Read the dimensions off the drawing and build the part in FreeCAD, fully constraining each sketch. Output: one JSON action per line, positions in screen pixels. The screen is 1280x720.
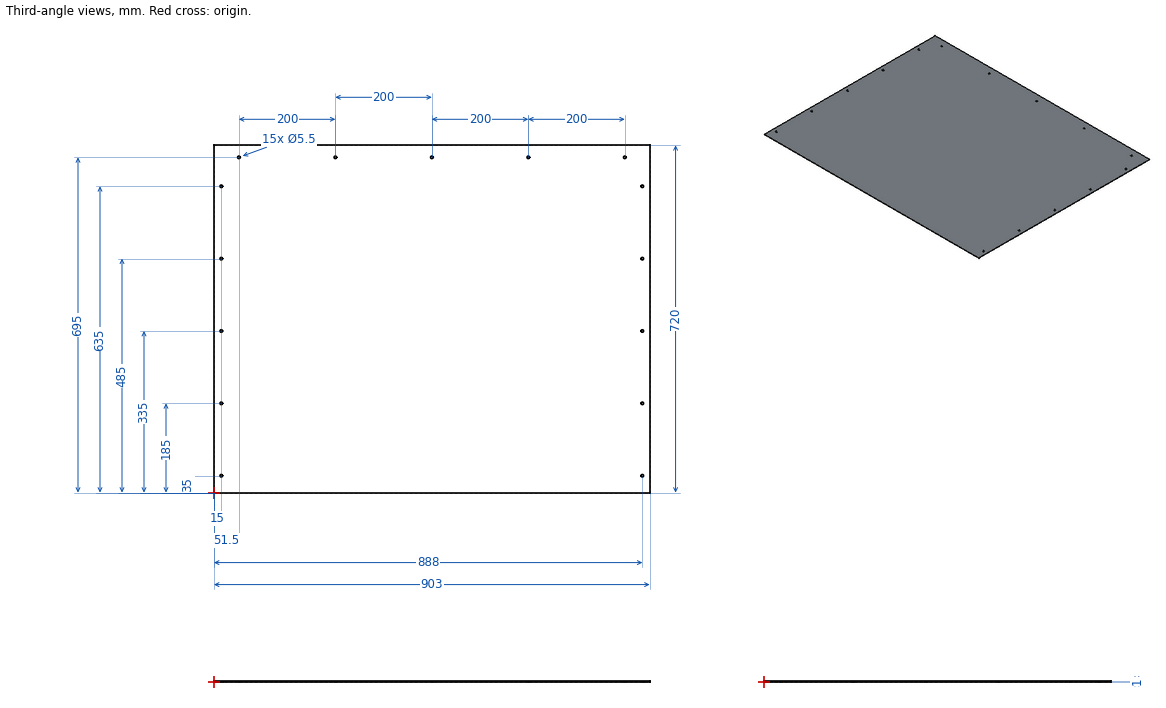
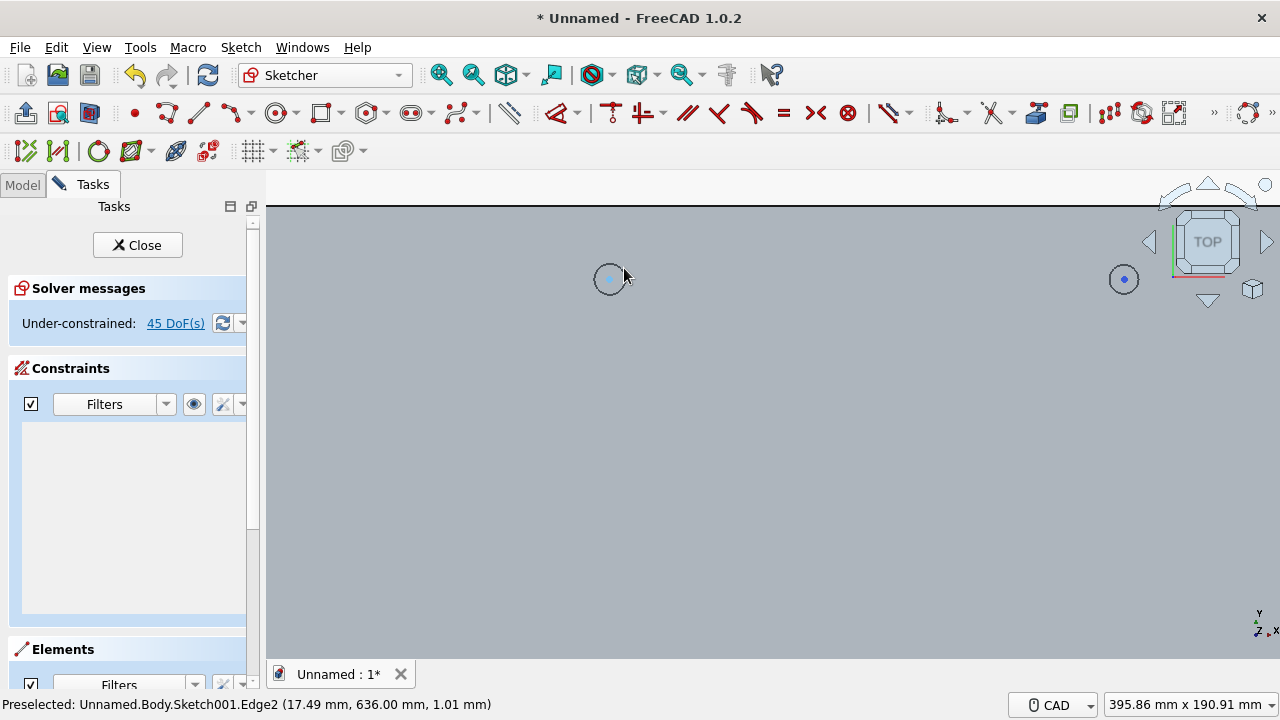
{"action": "left_click", "coordinate": [621, 268]}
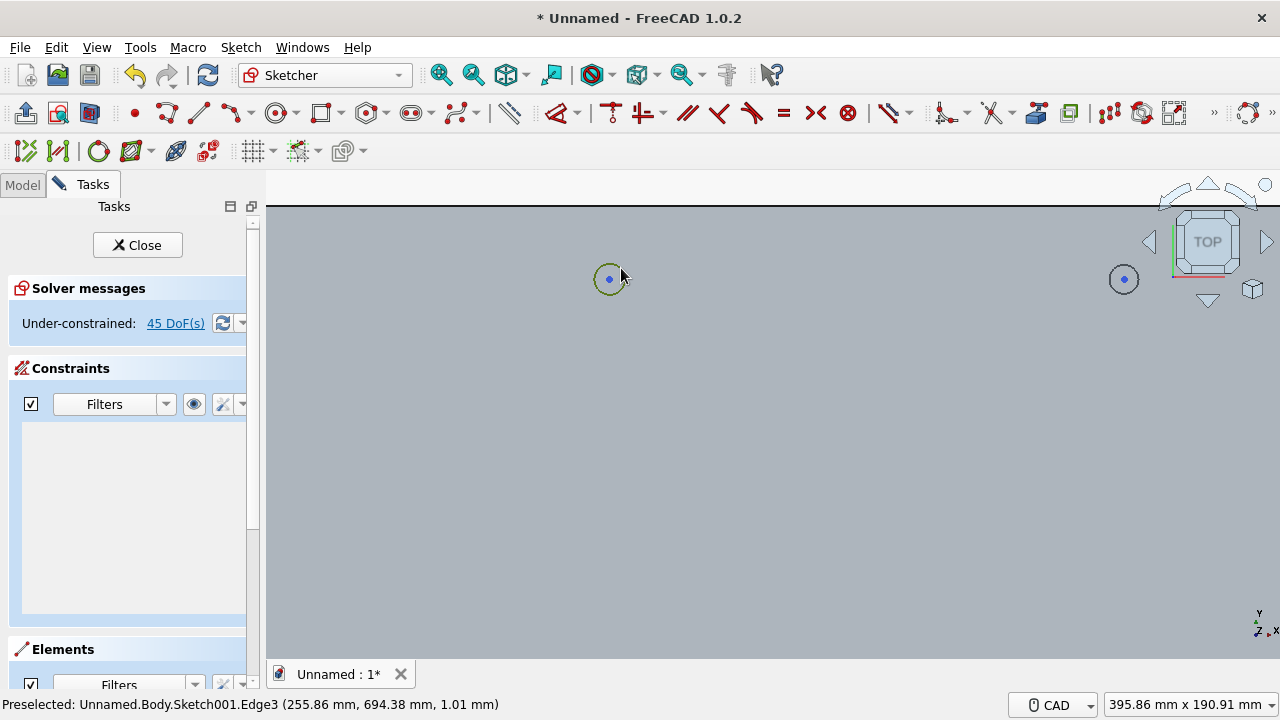
{"action": "left_click", "coordinate": [1114, 269]}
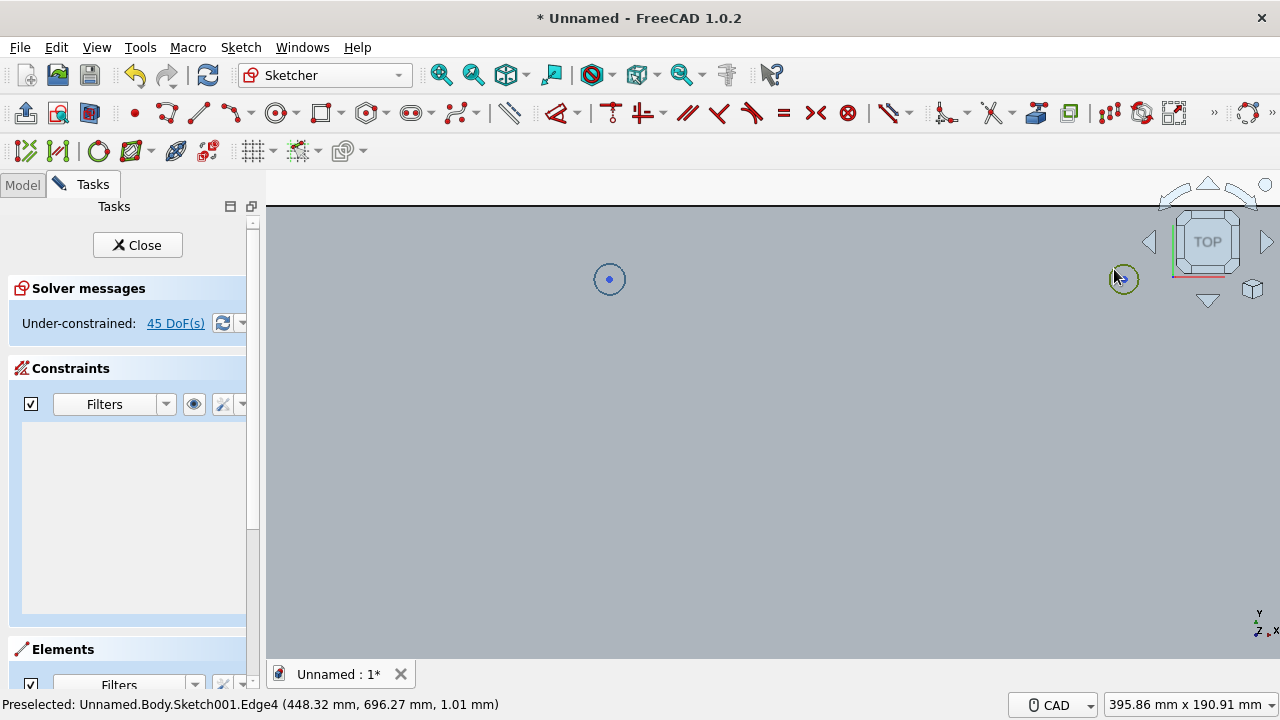
{"action": "scroll", "coordinate": [624, 267], "scroll_direction": "down", "scroll_amount": 9}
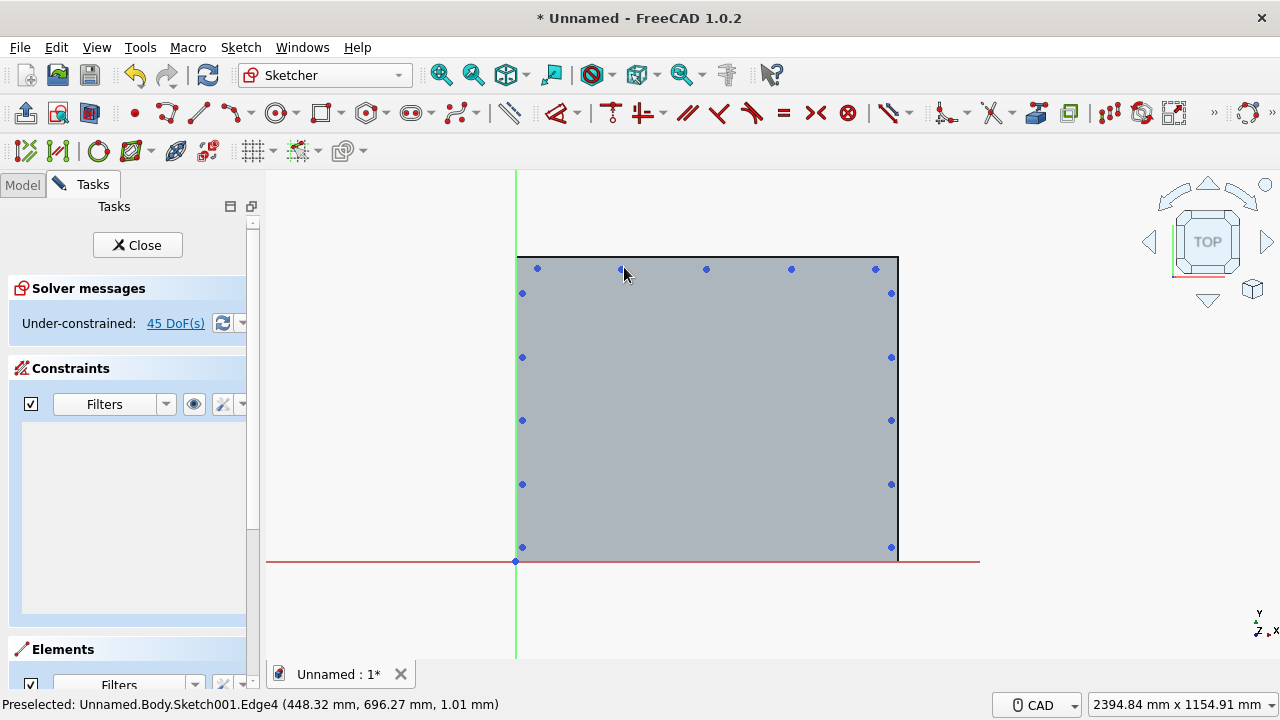
{"action": "scroll", "coordinate": [794, 268], "scroll_direction": "up", "scroll_amount": 9}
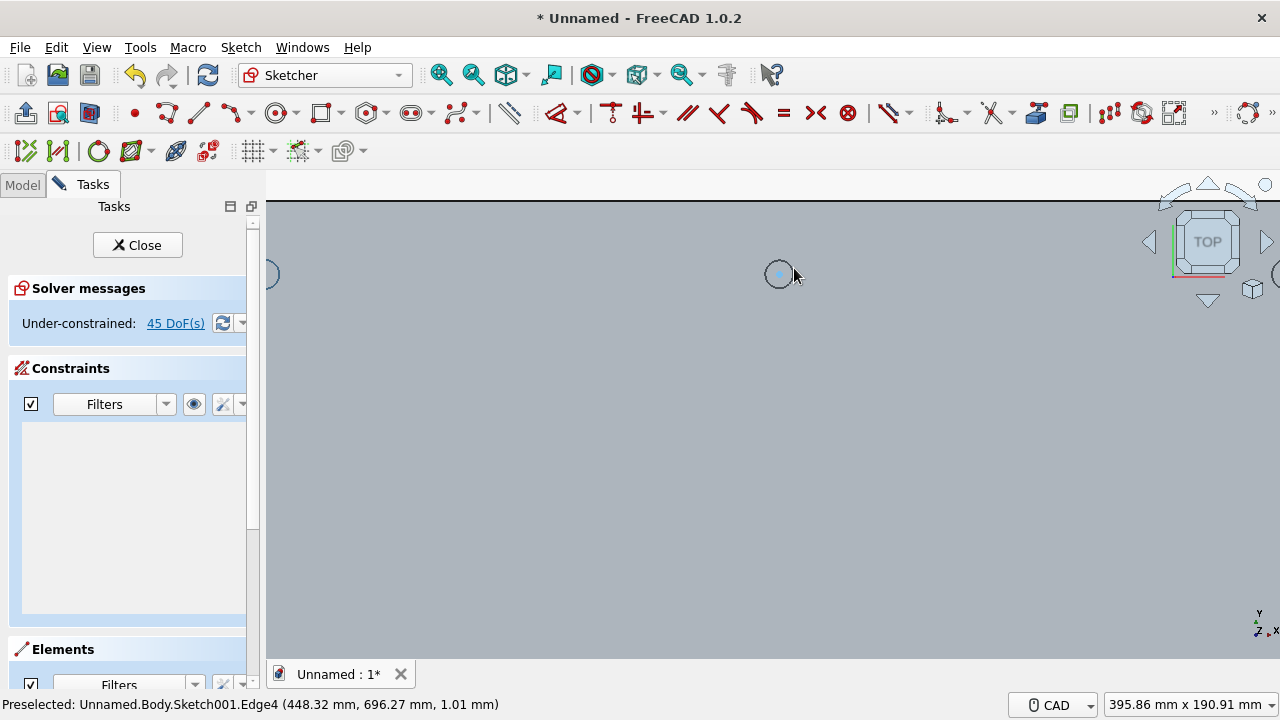
{"action": "left_click", "coordinate": [789, 264]}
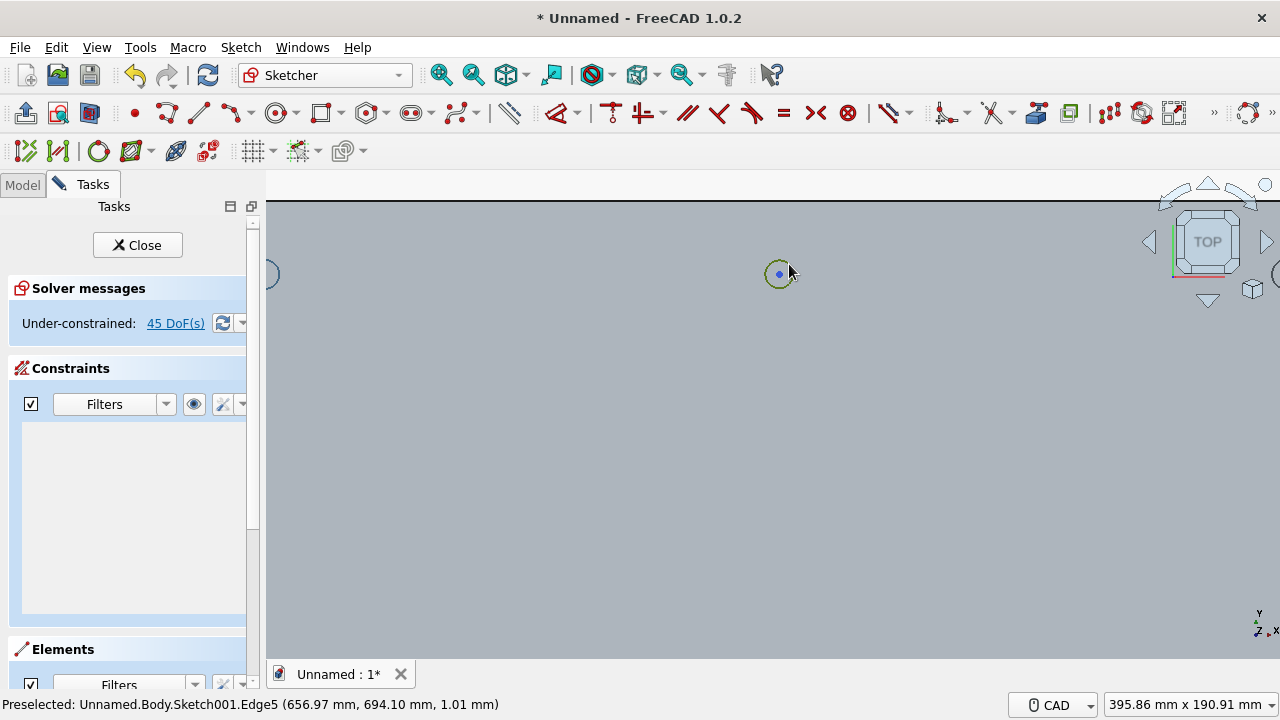
{"action": "scroll", "coordinate": [795, 268], "scroll_direction": "down", "scroll_amount": 9}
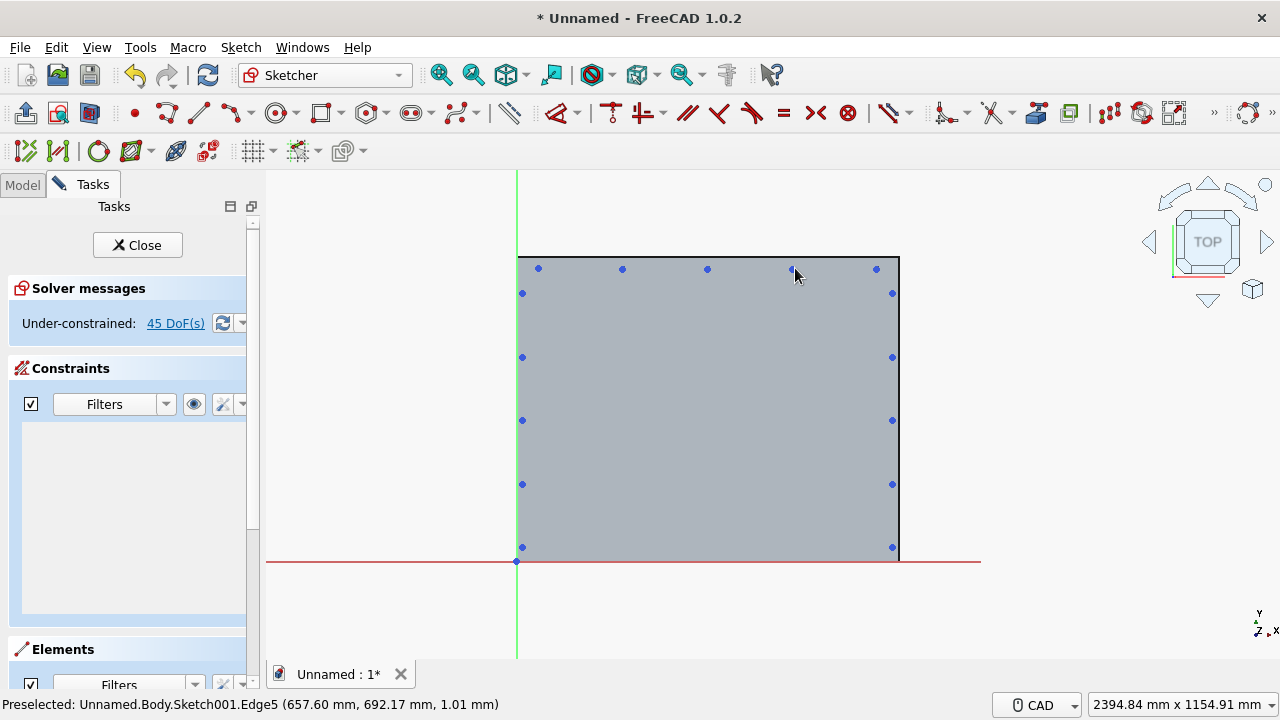
{"action": "scroll", "coordinate": [879, 267], "scroll_direction": "up", "scroll_amount": 9}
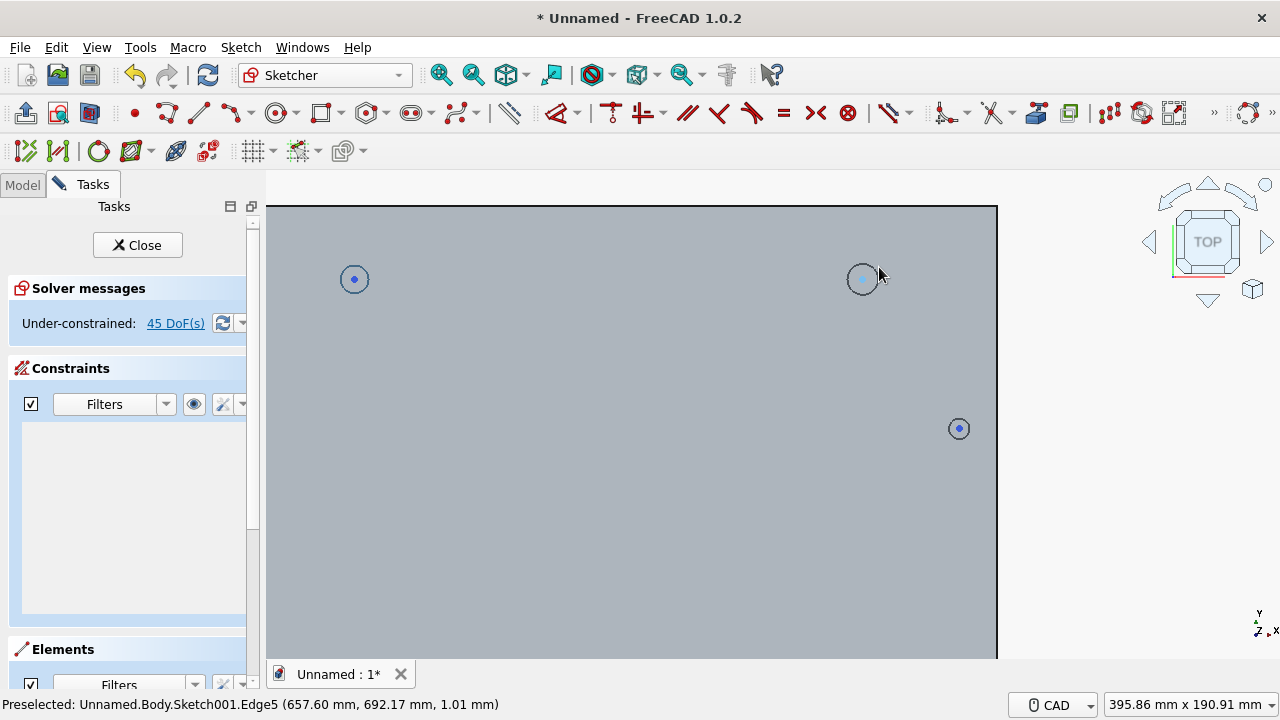
{"action": "left_click", "coordinate": [874, 268]}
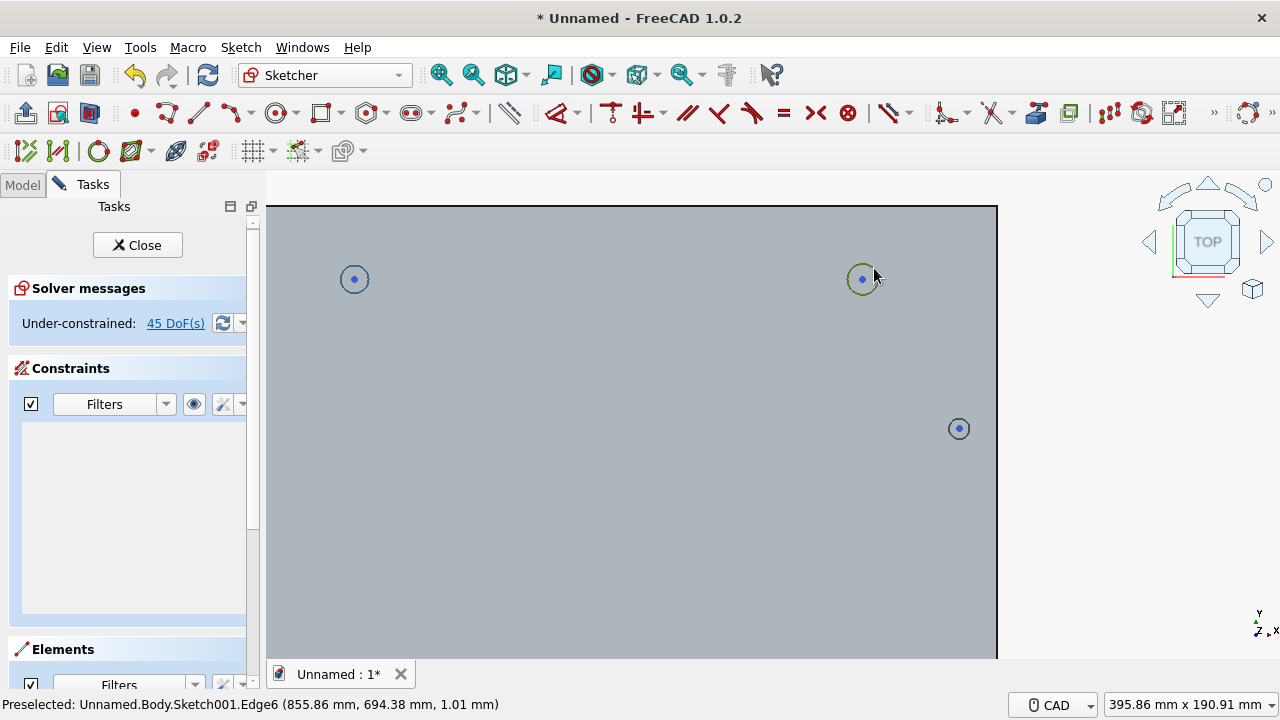
{"action": "scroll", "coordinate": [879, 267], "scroll_direction": "down", "scroll_amount": 9}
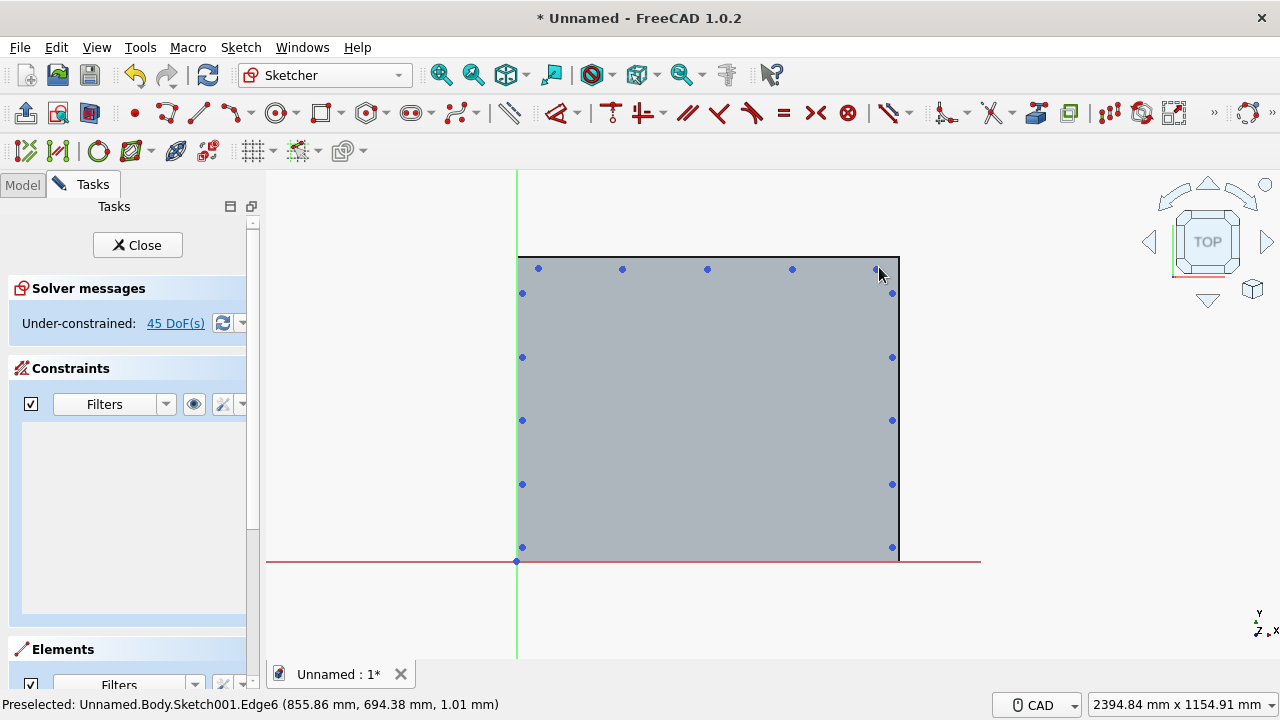
{"action": "scroll", "coordinate": [524, 356], "scroll_direction": "up", "scroll_amount": 11}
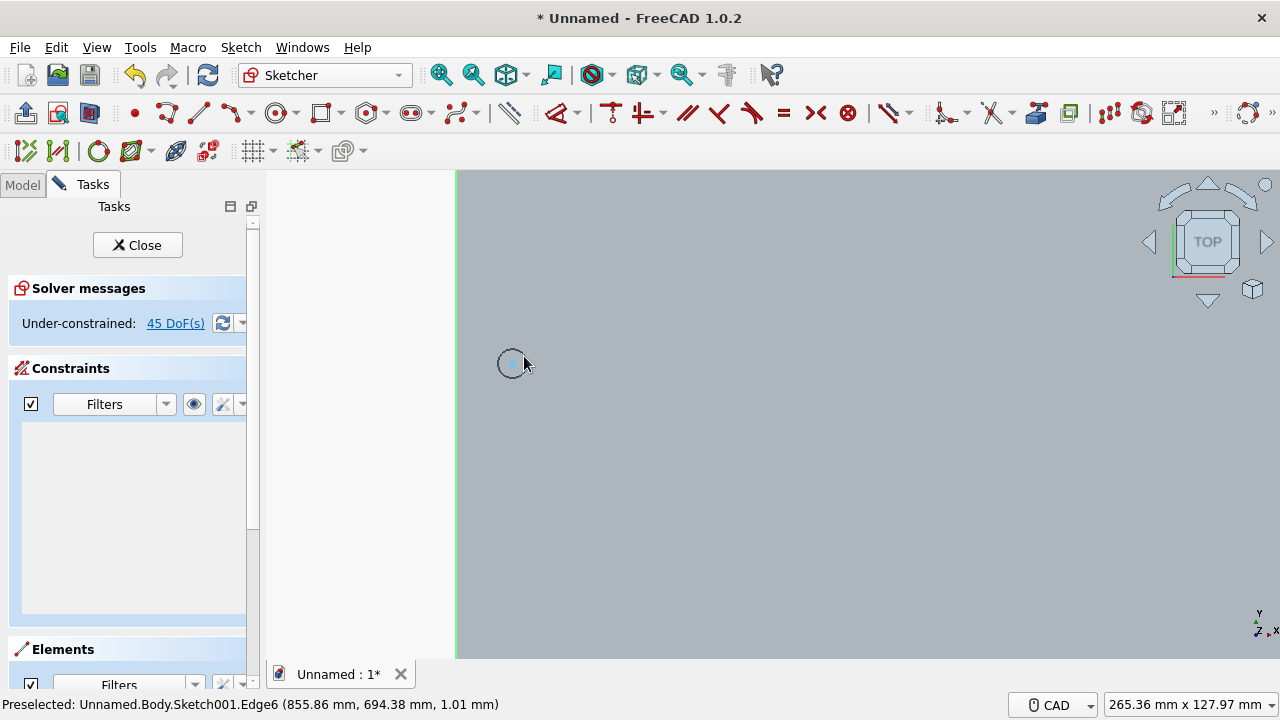
{"action": "left_click", "coordinate": [523, 353]}